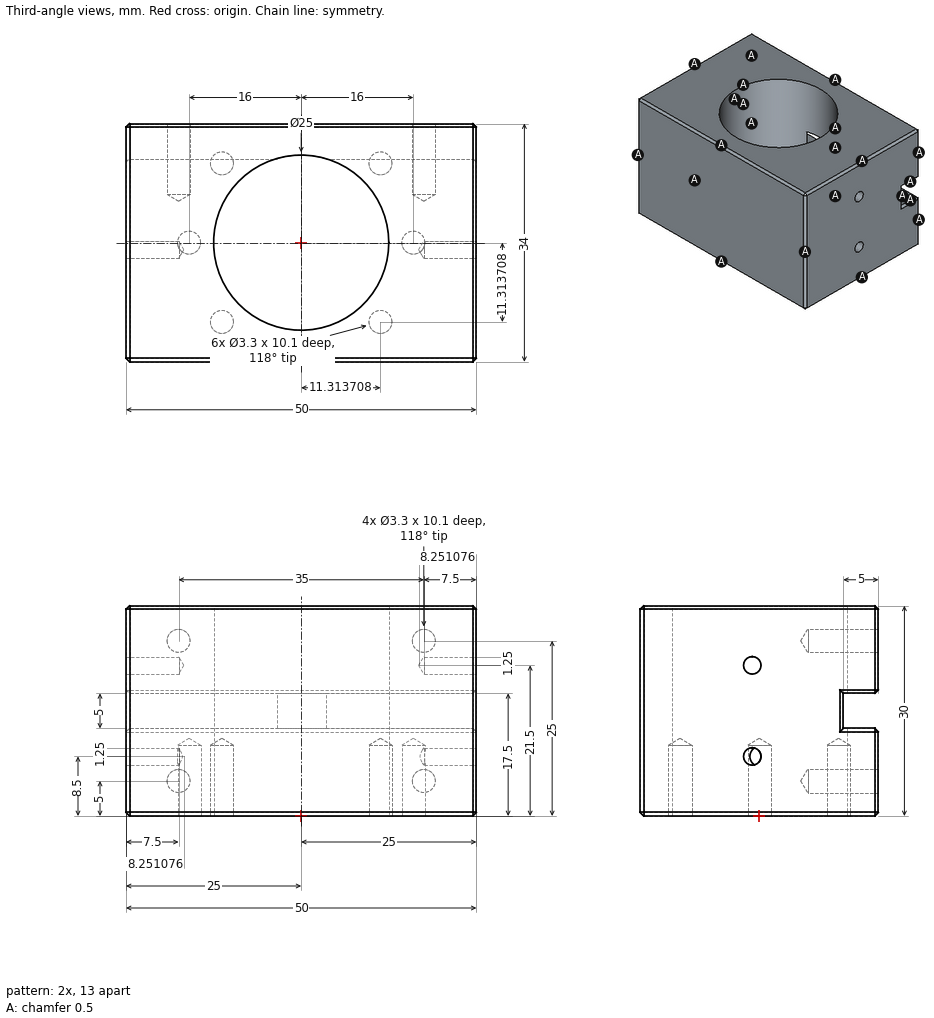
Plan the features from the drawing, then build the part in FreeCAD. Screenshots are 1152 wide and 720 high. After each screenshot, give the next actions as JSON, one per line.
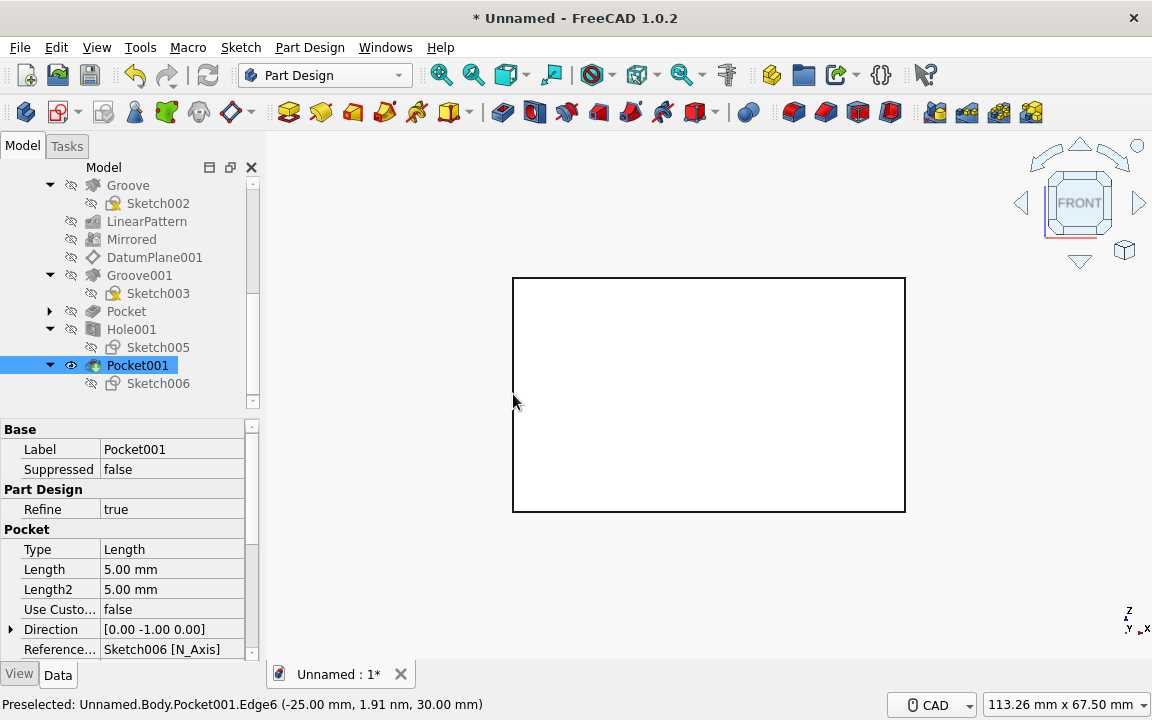
{"action": "key", "text": "3"}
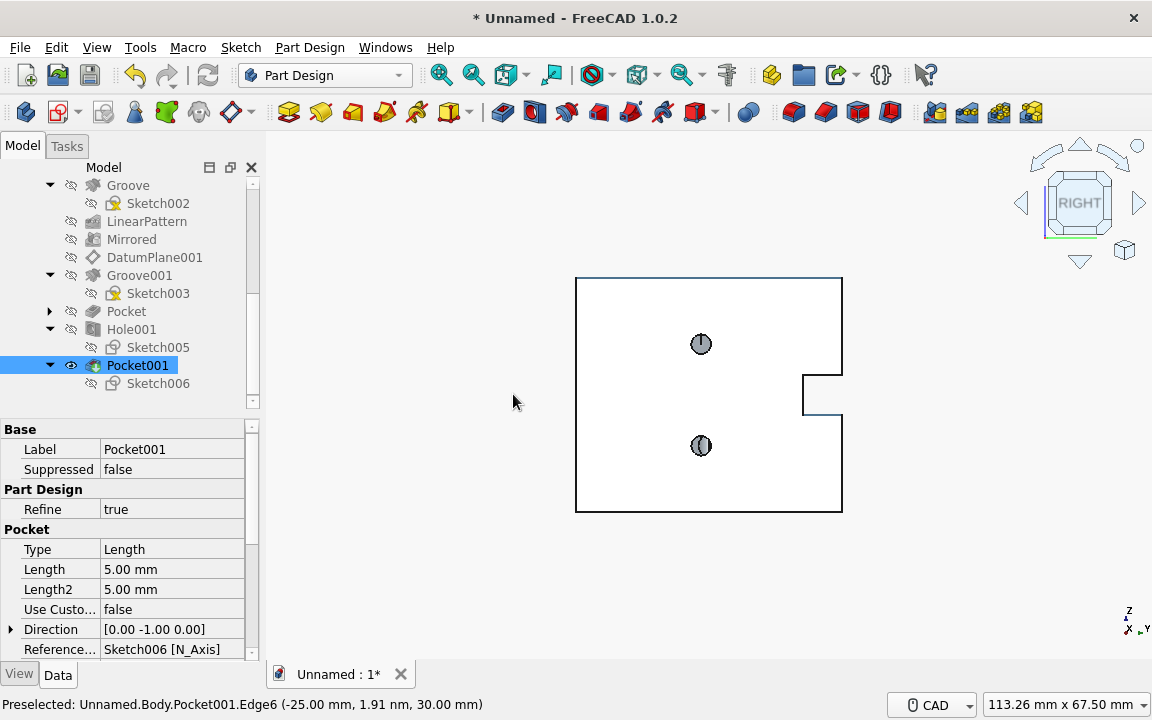
{"action": "left_click", "coordinate": [442, 76]}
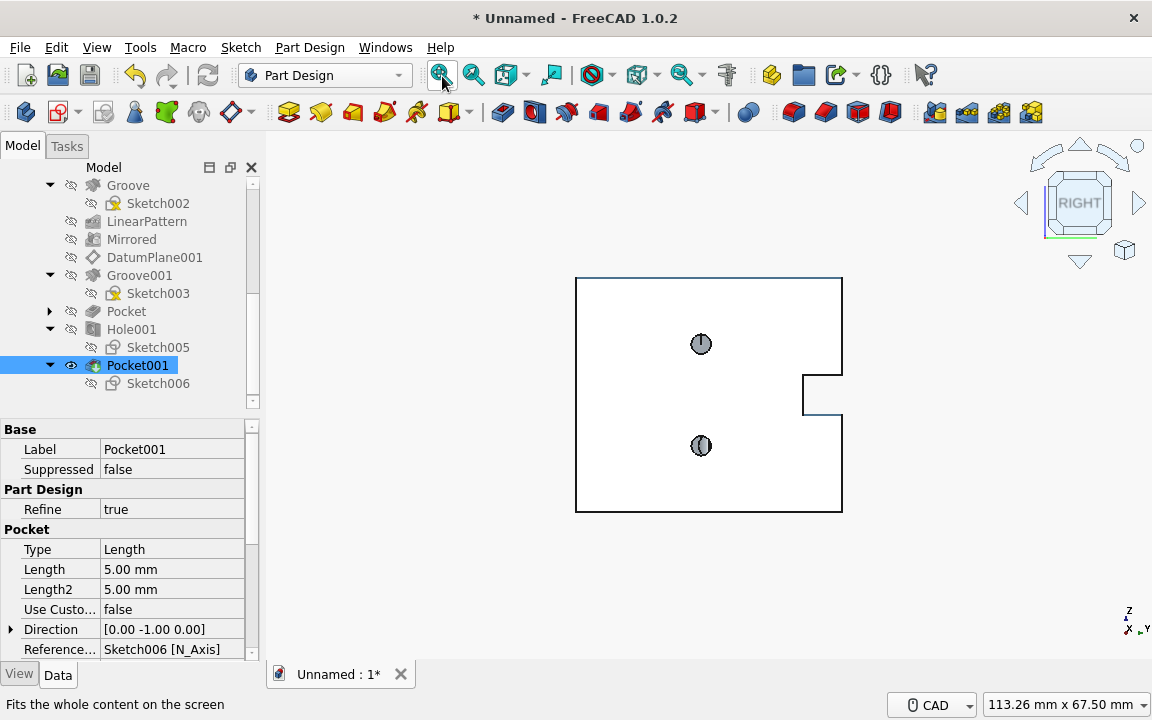
{"action": "left_click", "coordinate": [709, 511], "text": "ctrl"}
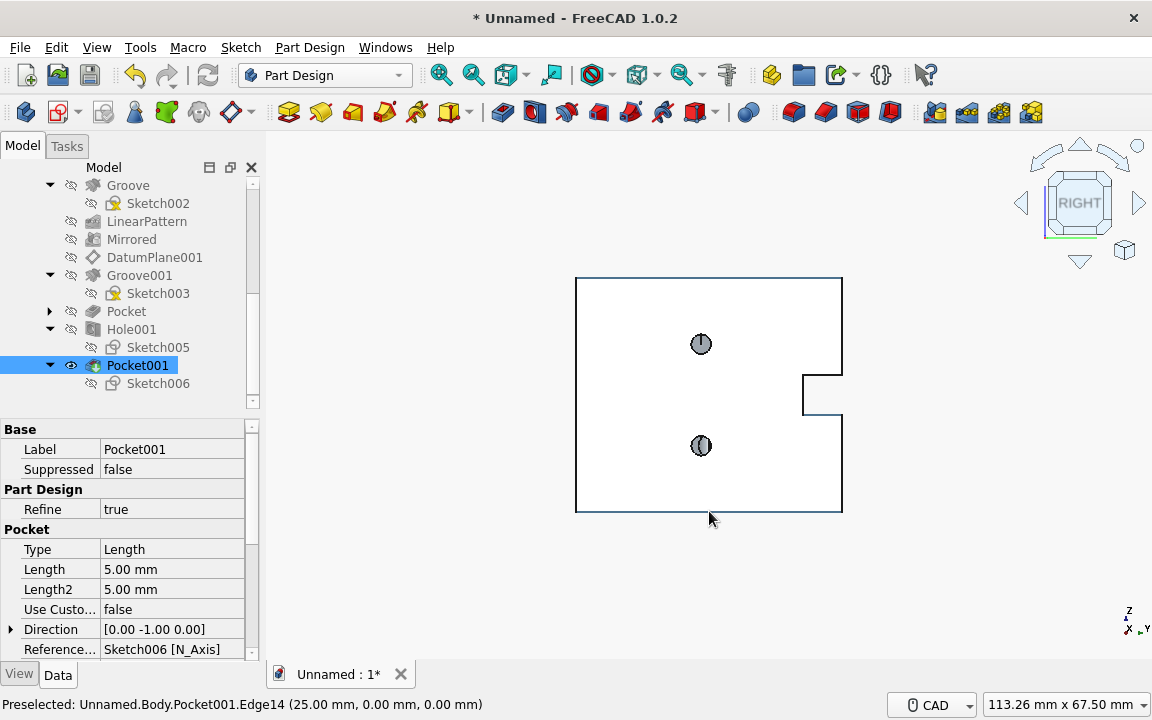
{"action": "left_click", "coordinate": [842, 326], "text": "ctrl"}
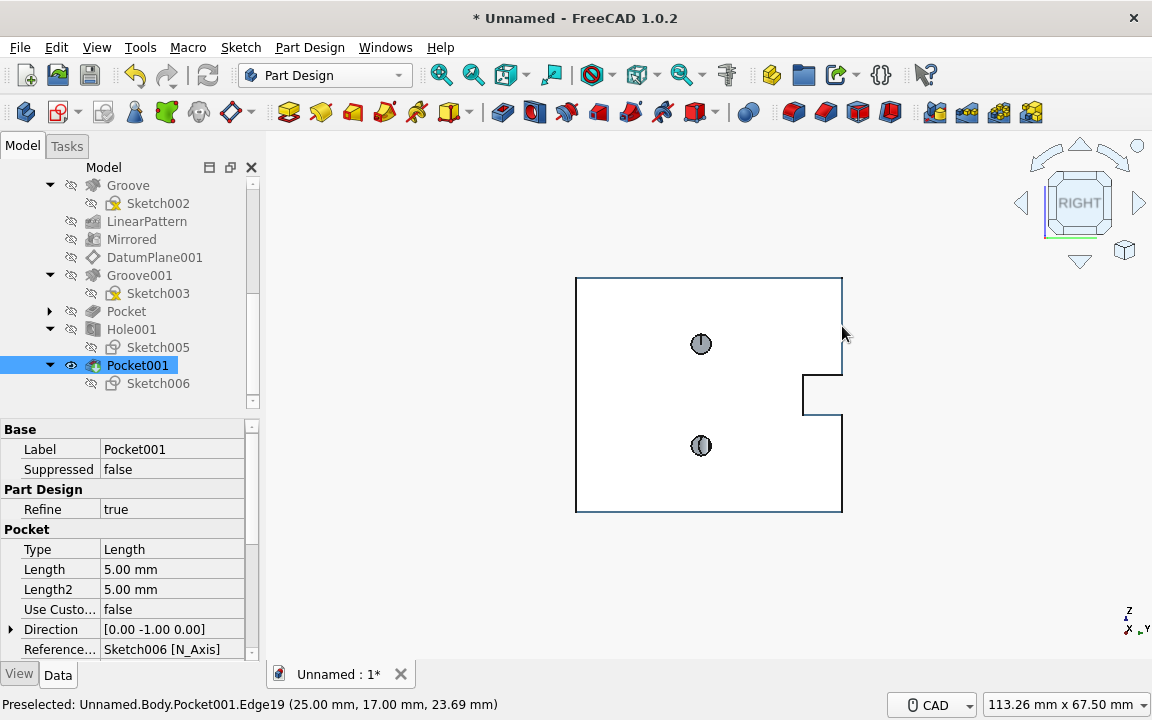
{"action": "left_click", "coordinate": [842, 462], "text": "ctrl"}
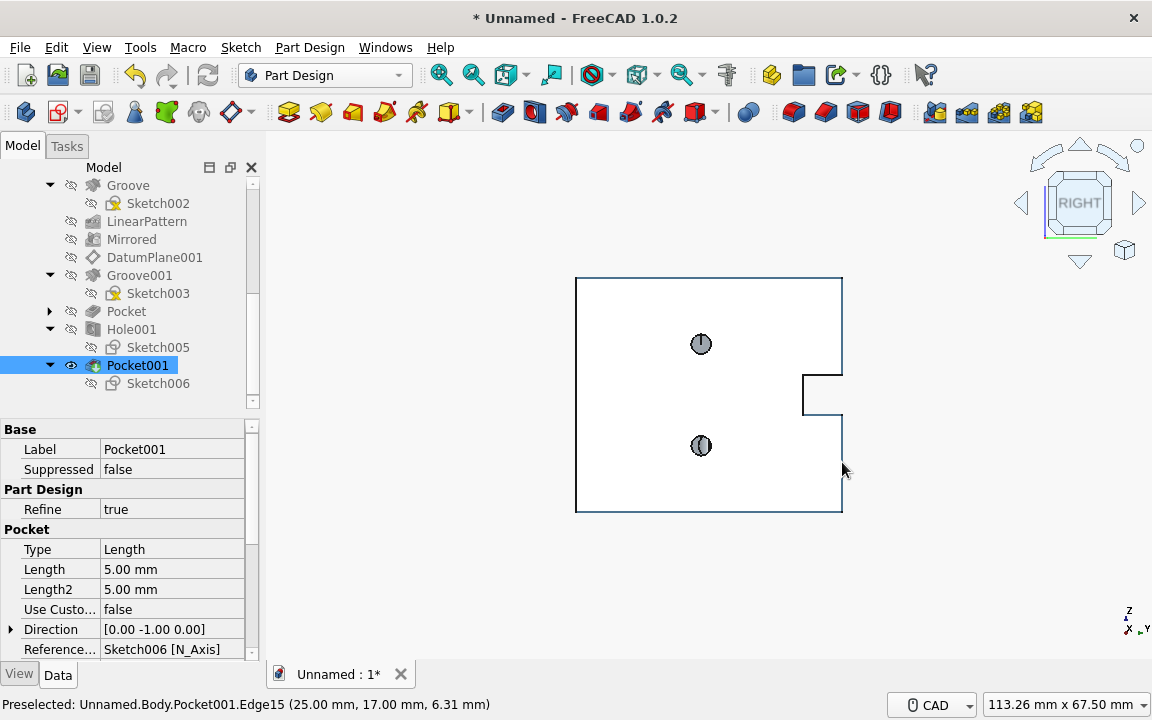
{"action": "left_click", "coordinate": [822, 374], "text": "ctrl"}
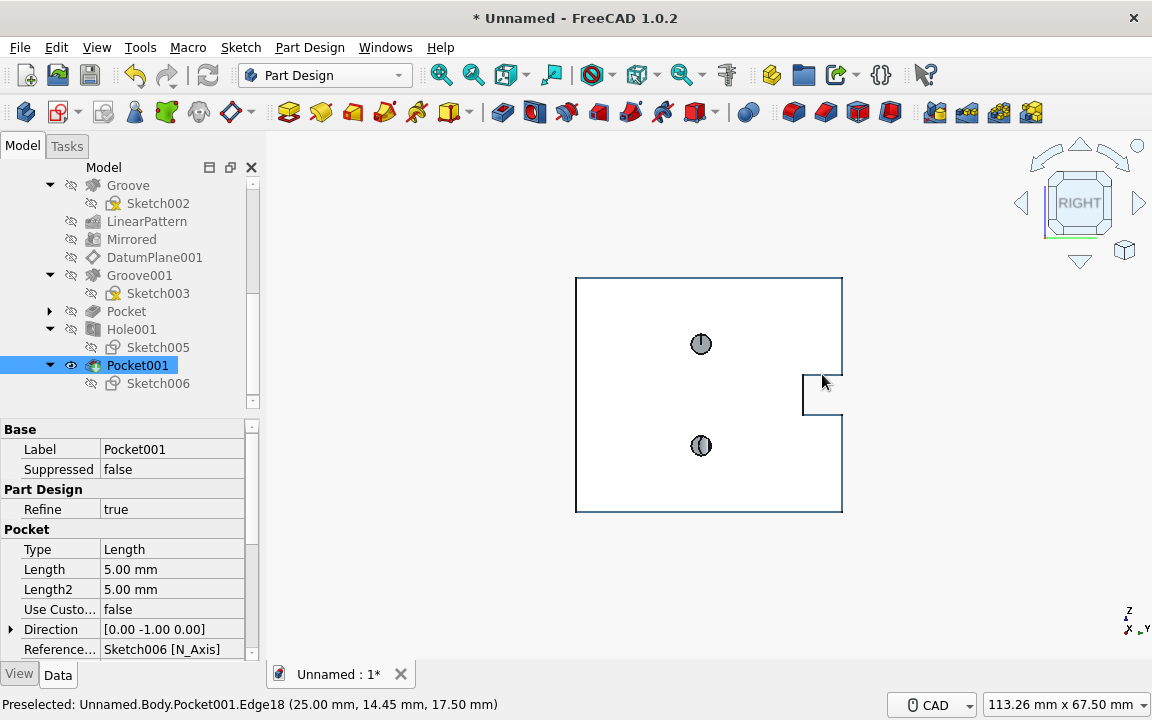
{"action": "left_click", "coordinate": [803, 394], "text": "ctrl"}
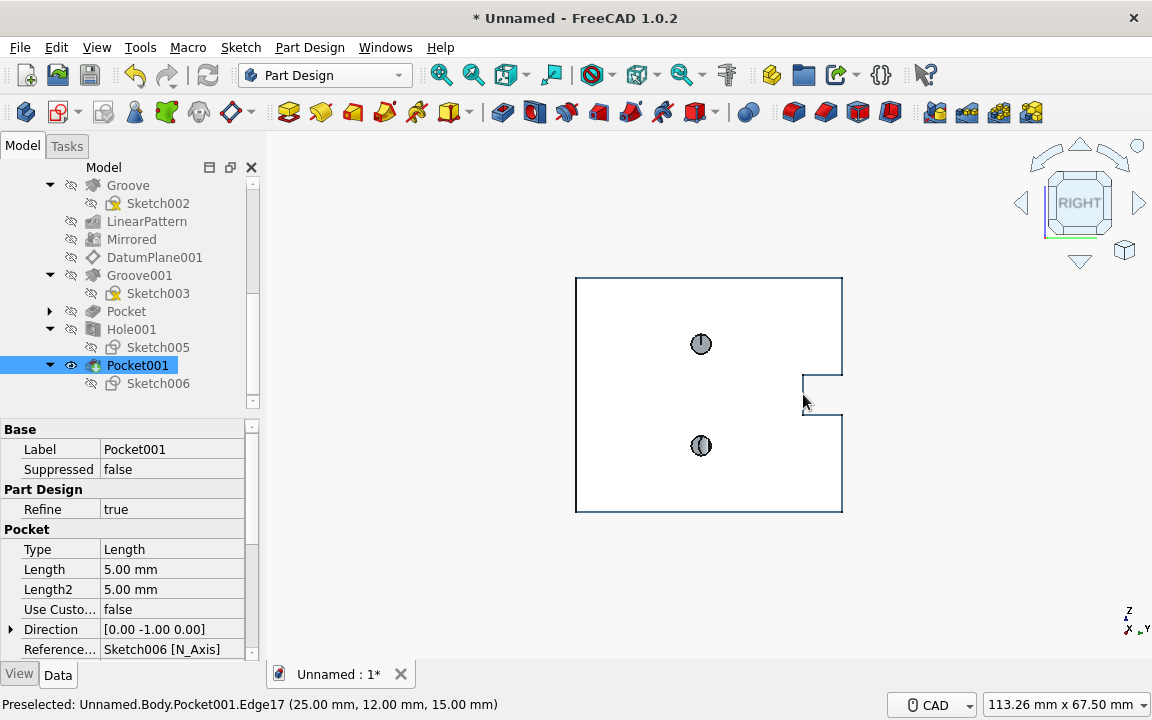
{"action": "key", "text": "5"}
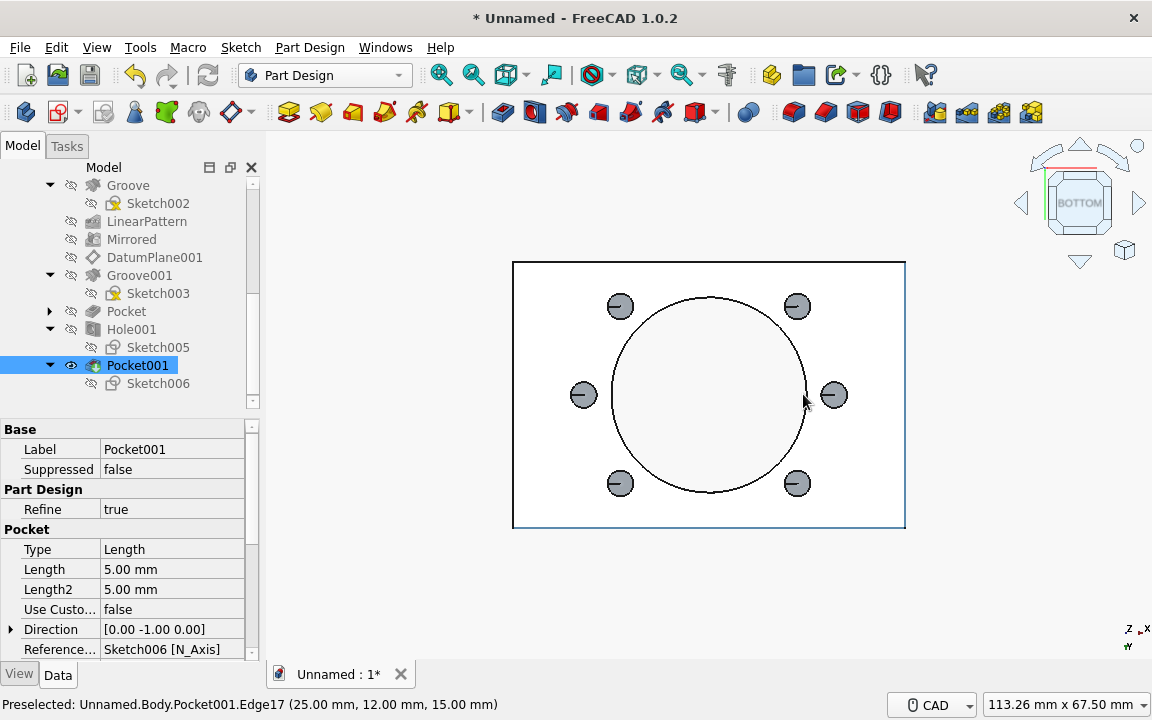
{"action": "left_click", "coordinate": [513, 394], "text": "ctrl"}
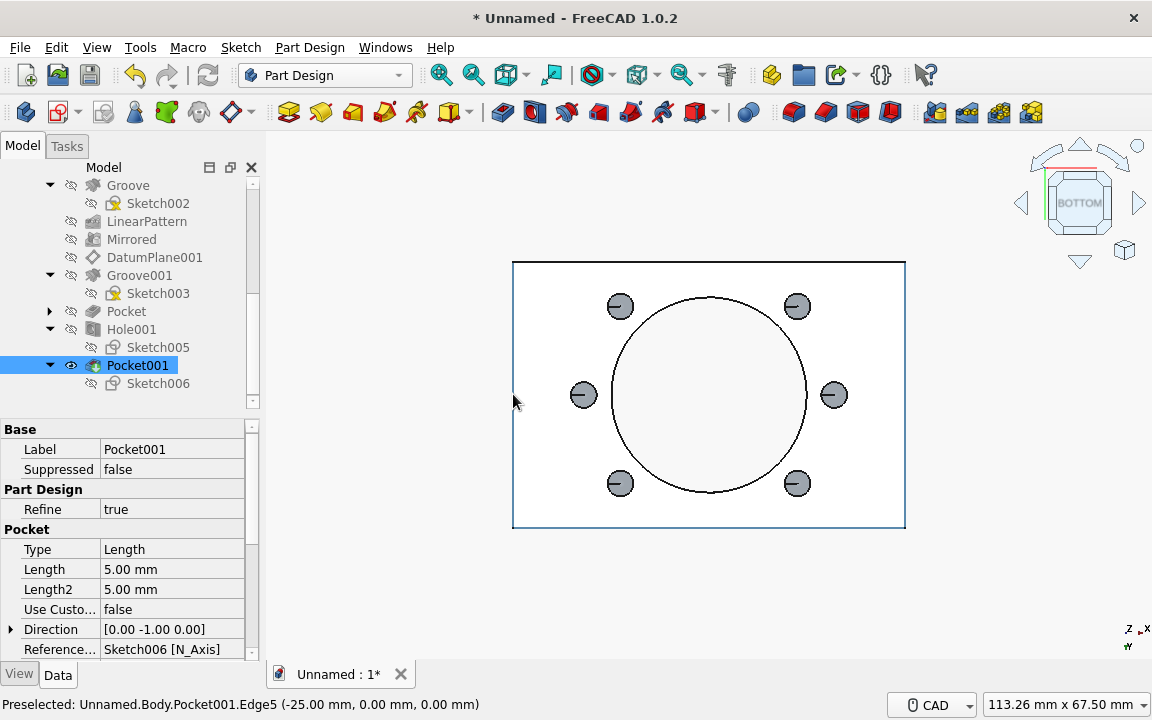
{"action": "key", "text": "4"}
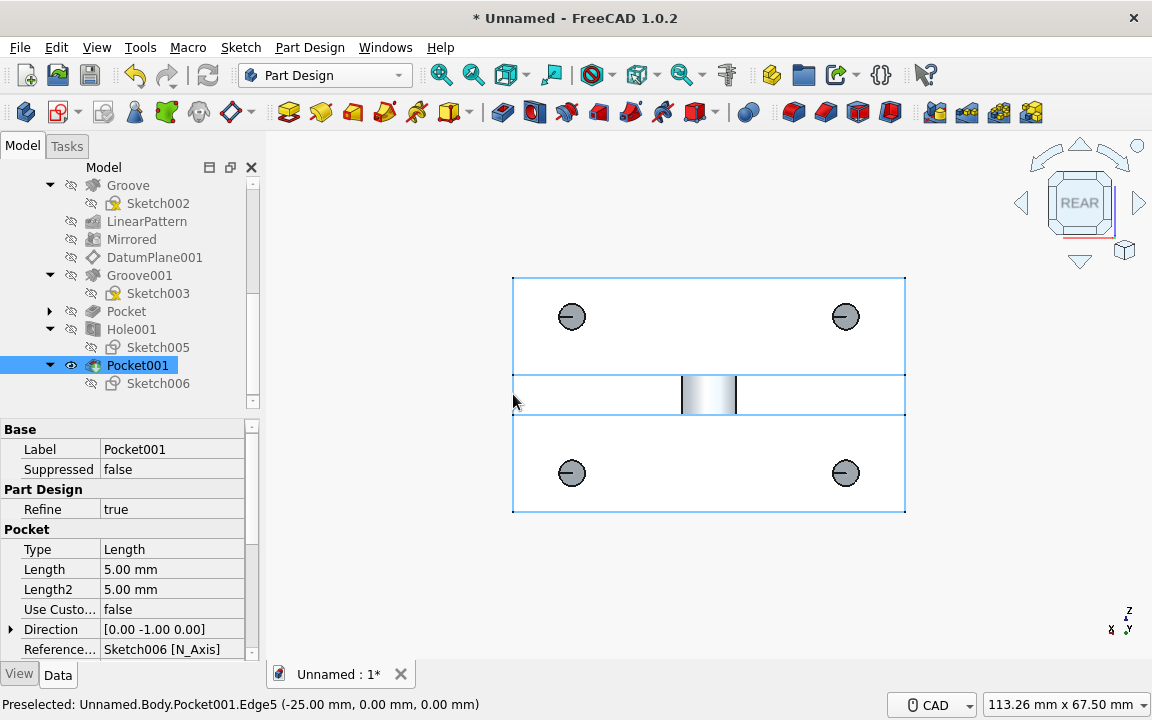
{"action": "left_click", "coordinate": [442, 76]}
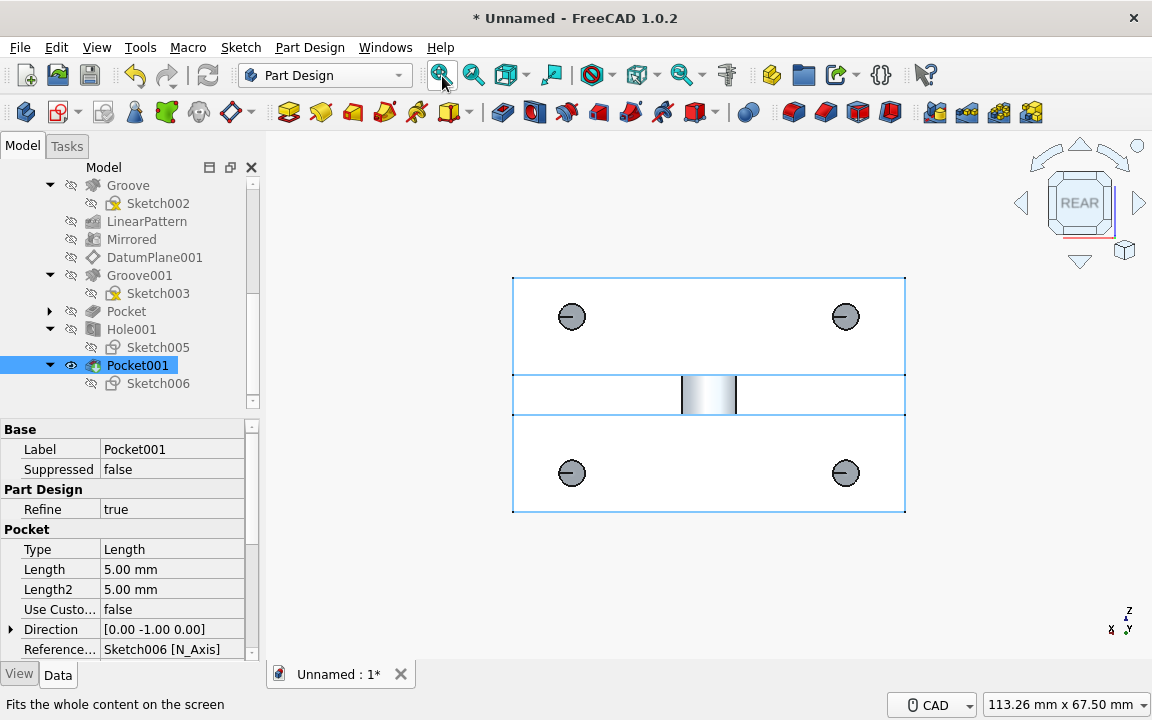
{"action": "key", "text": "6"}